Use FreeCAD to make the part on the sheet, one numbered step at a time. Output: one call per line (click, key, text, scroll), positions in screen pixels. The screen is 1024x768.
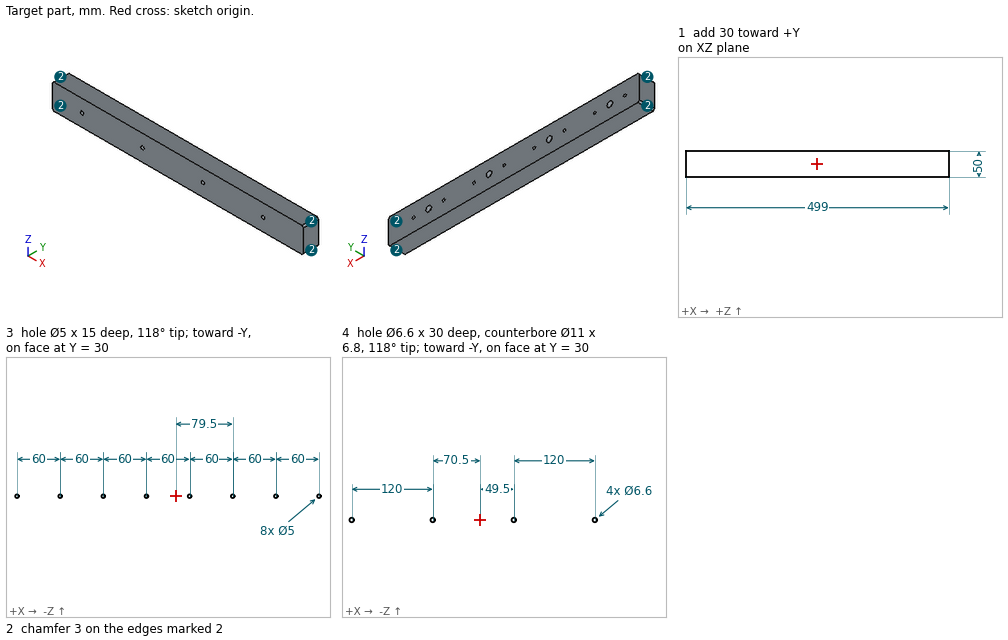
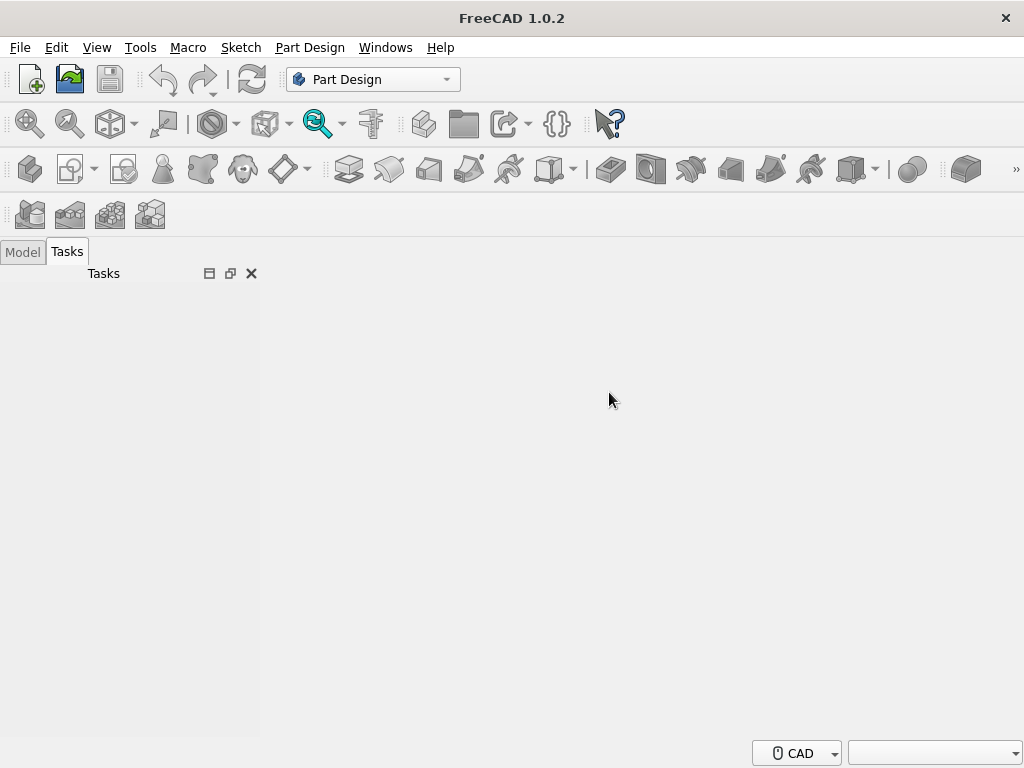
click(30, 80)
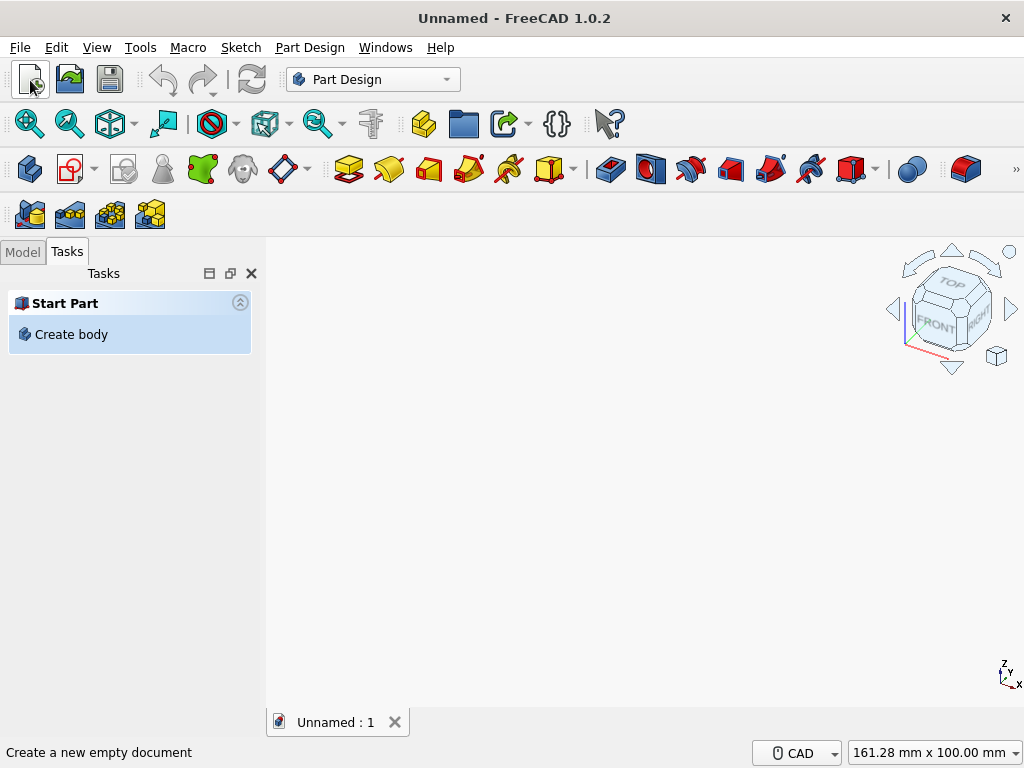
click(70, 170)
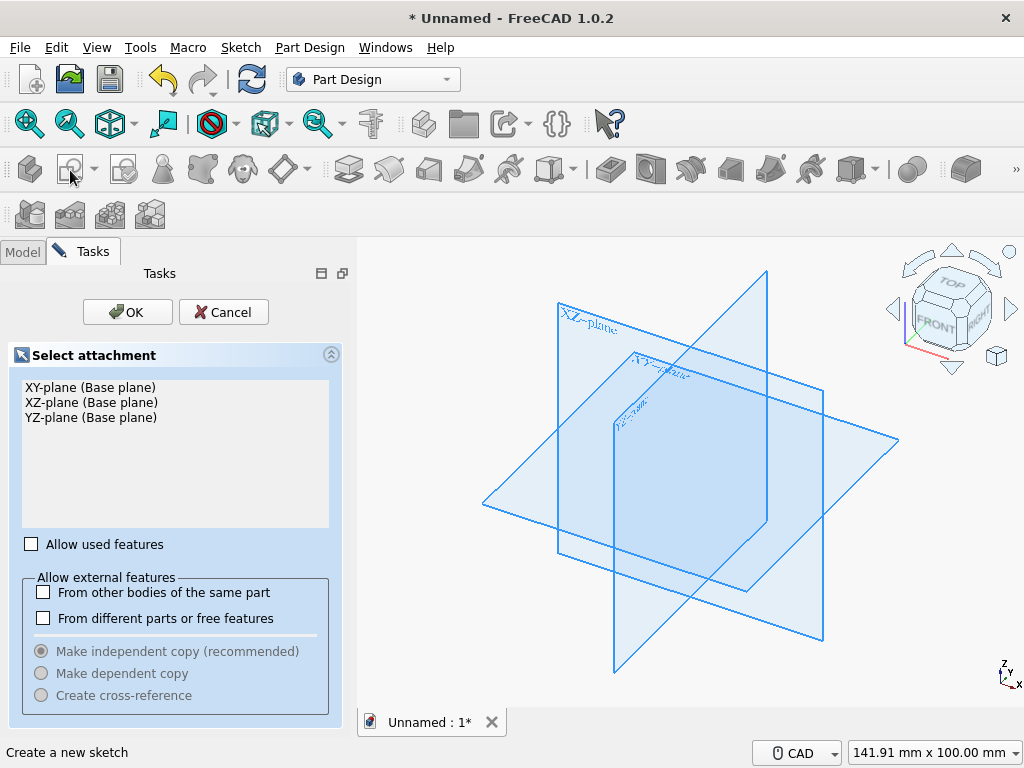
click(82, 402)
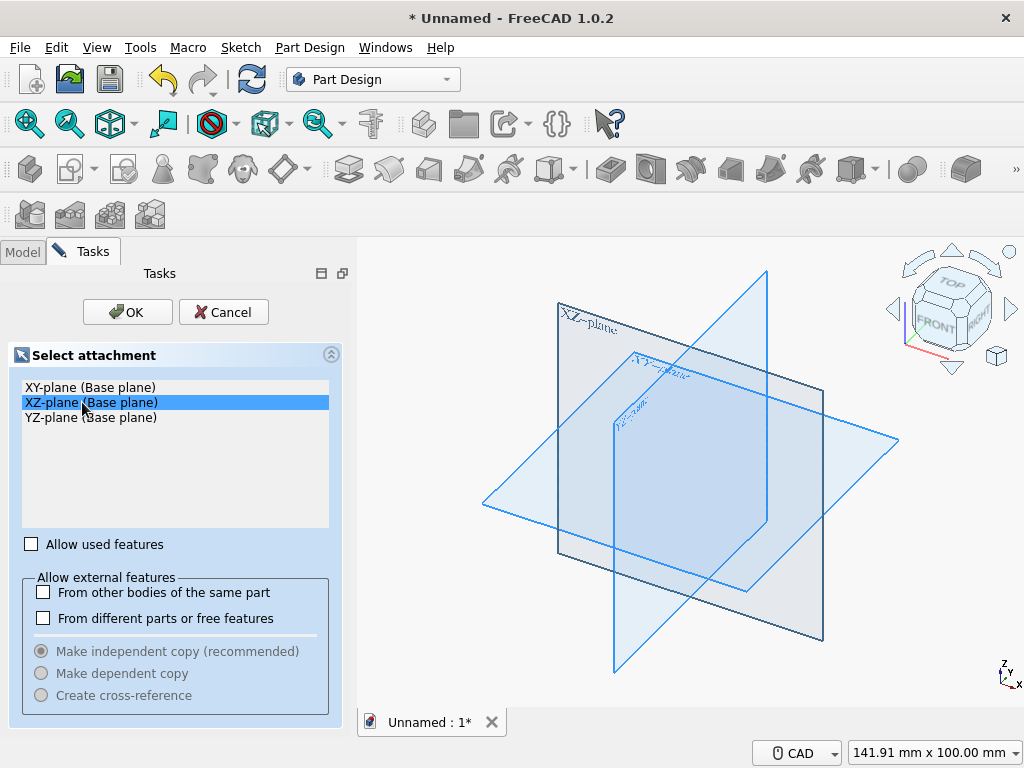
click(128, 312)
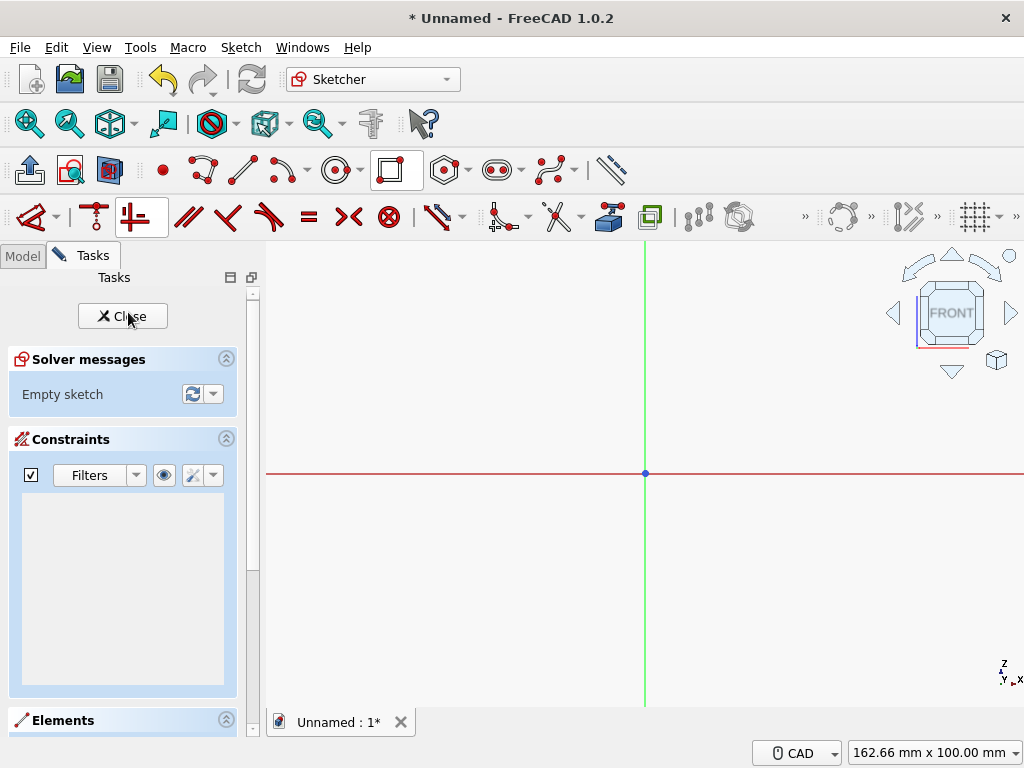
scroll(563, 474, down, 9)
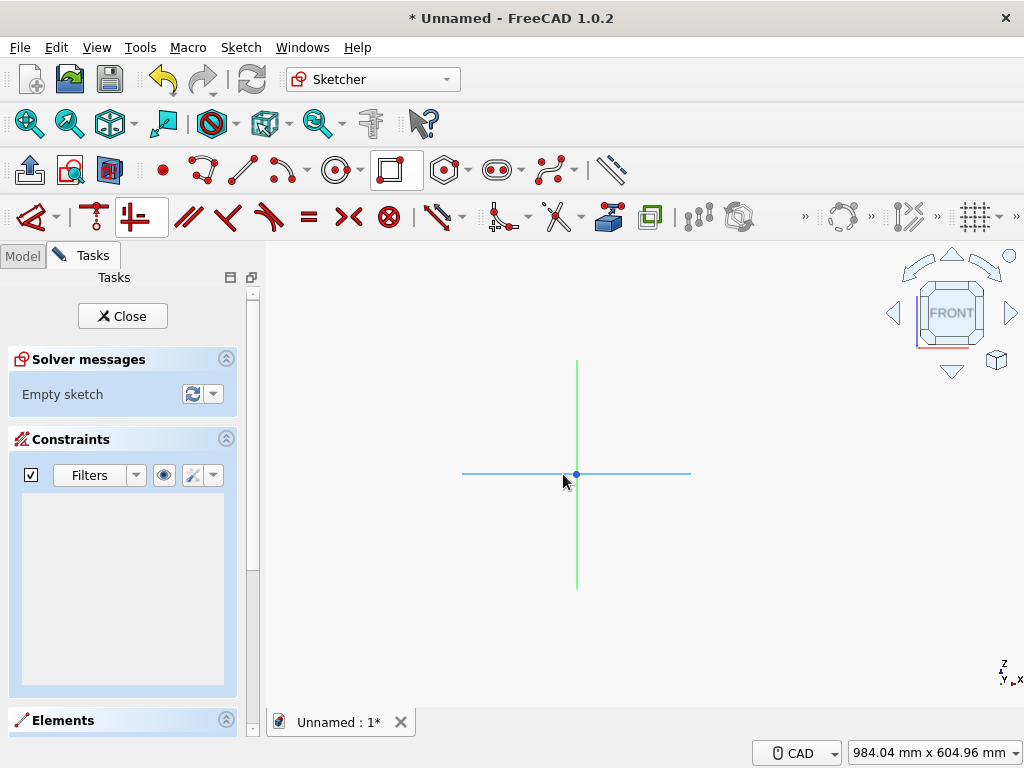
key(g)
key(v)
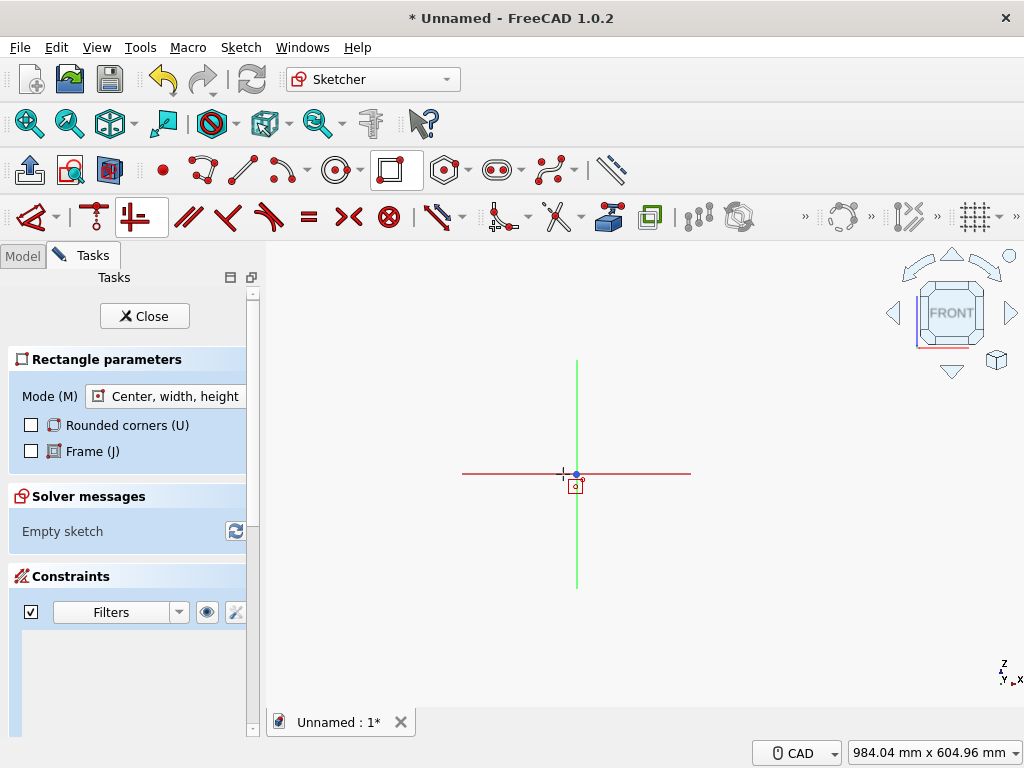
click(577, 474)
click(769, 455)
key(Escape)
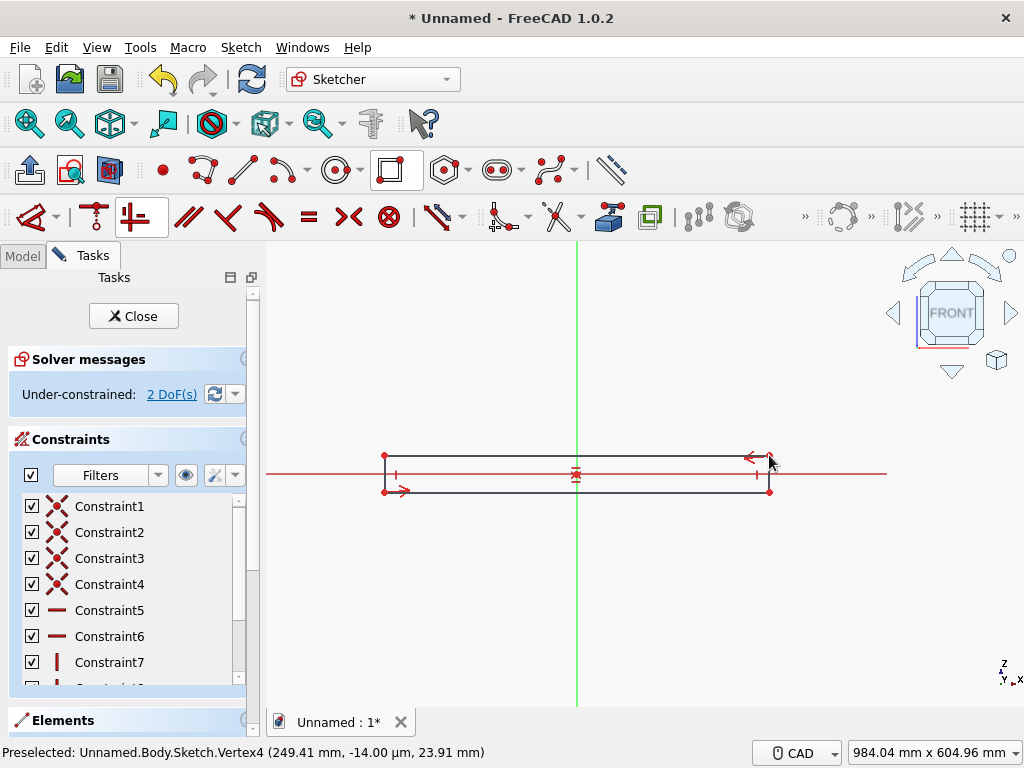
click(32, 218)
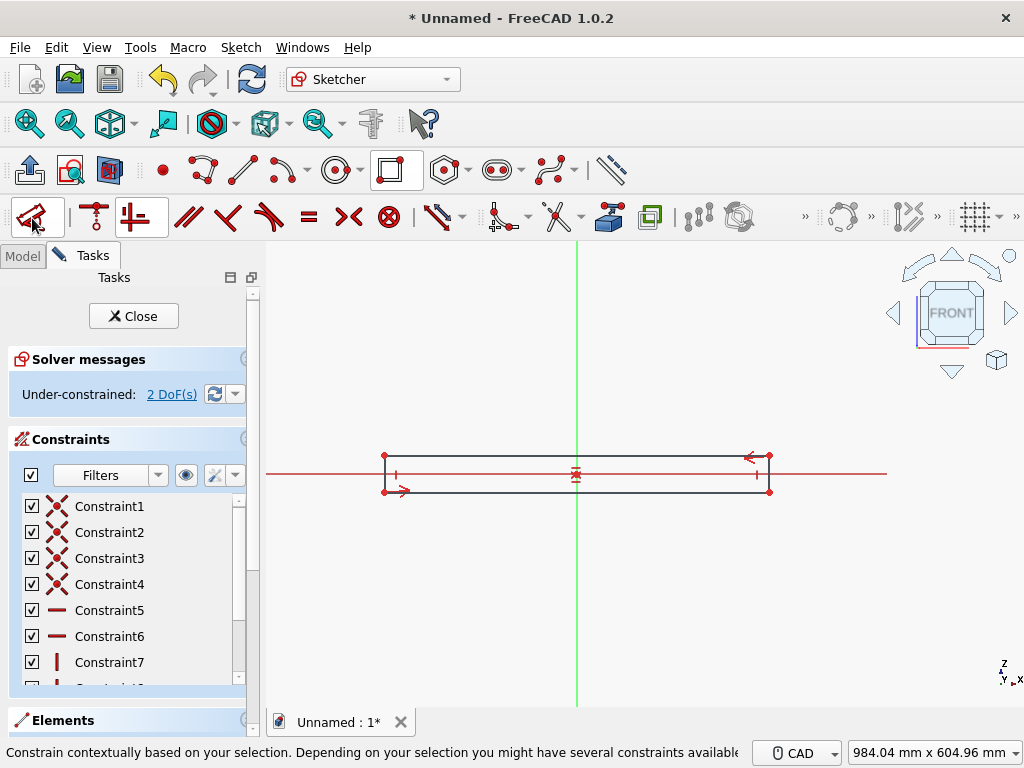
click(769, 478)
click(803, 466)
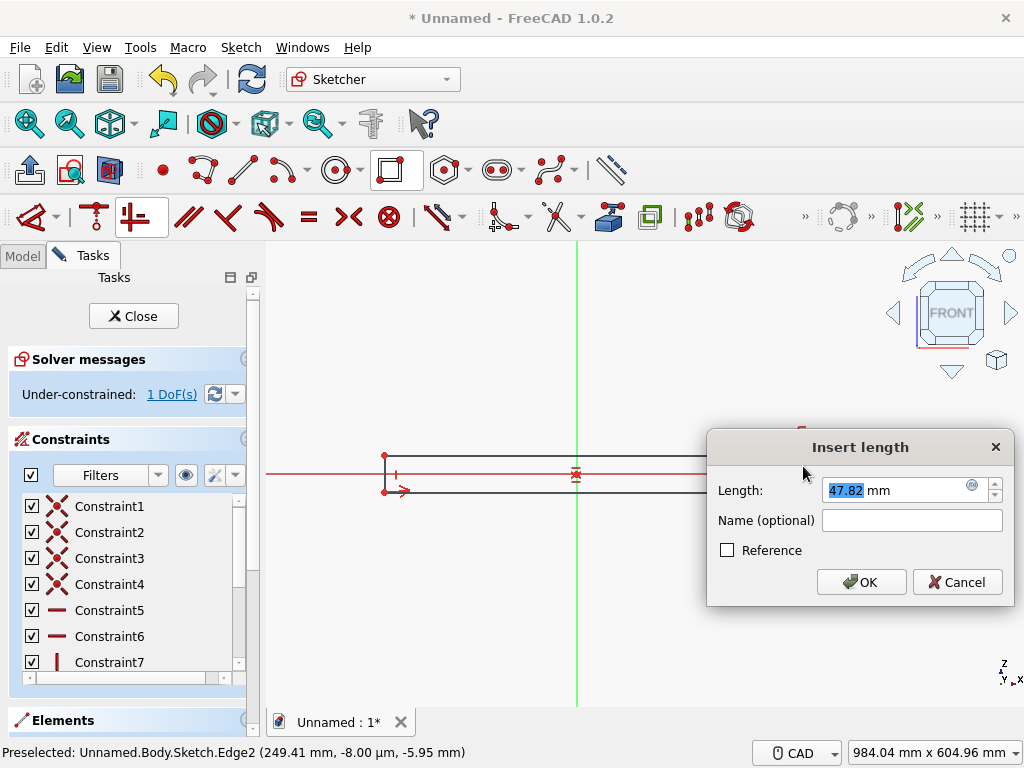
text(50)
key(Return)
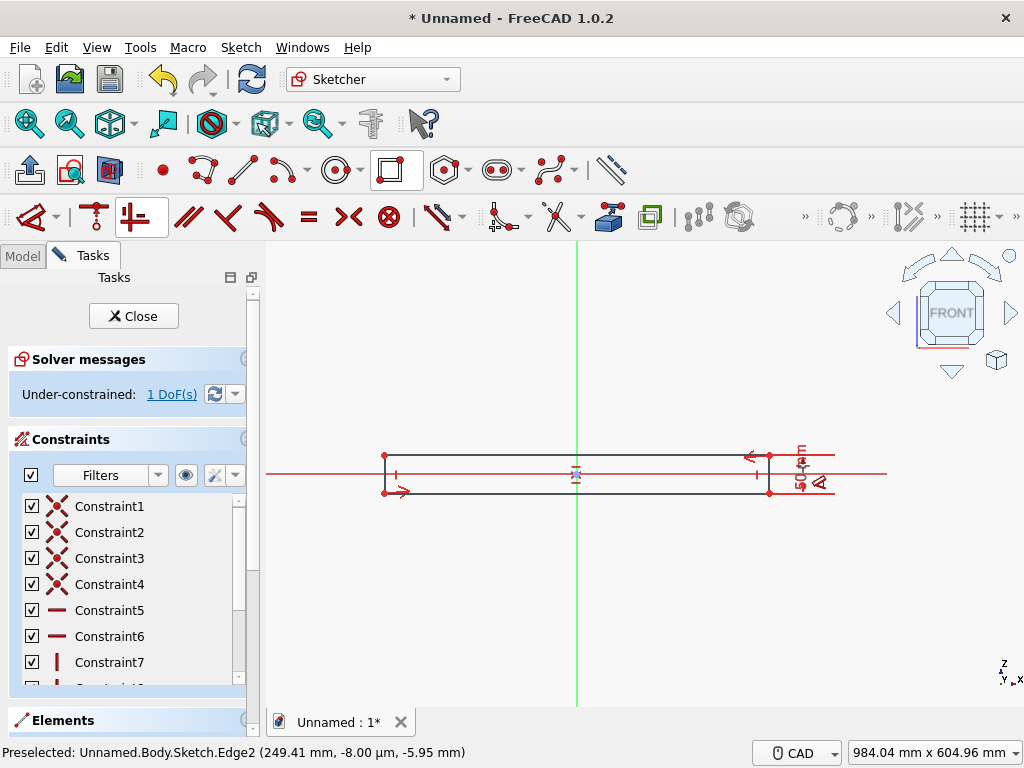
click(500, 494)
click(489, 528)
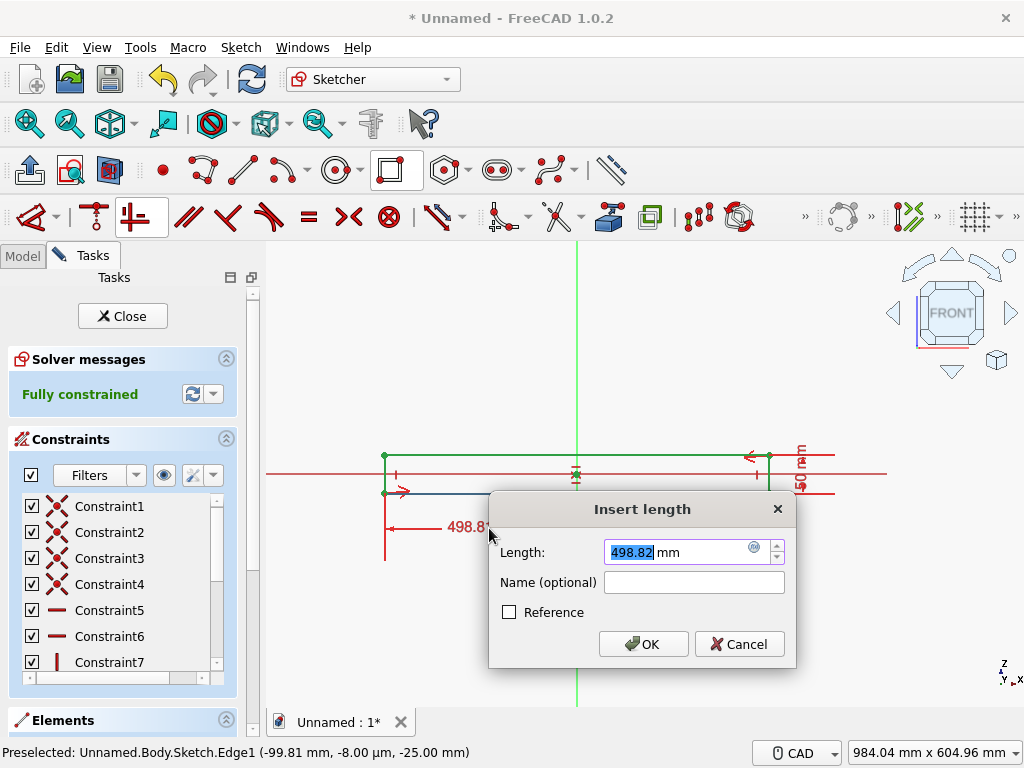
text(499)
key(Return)
key(Escape)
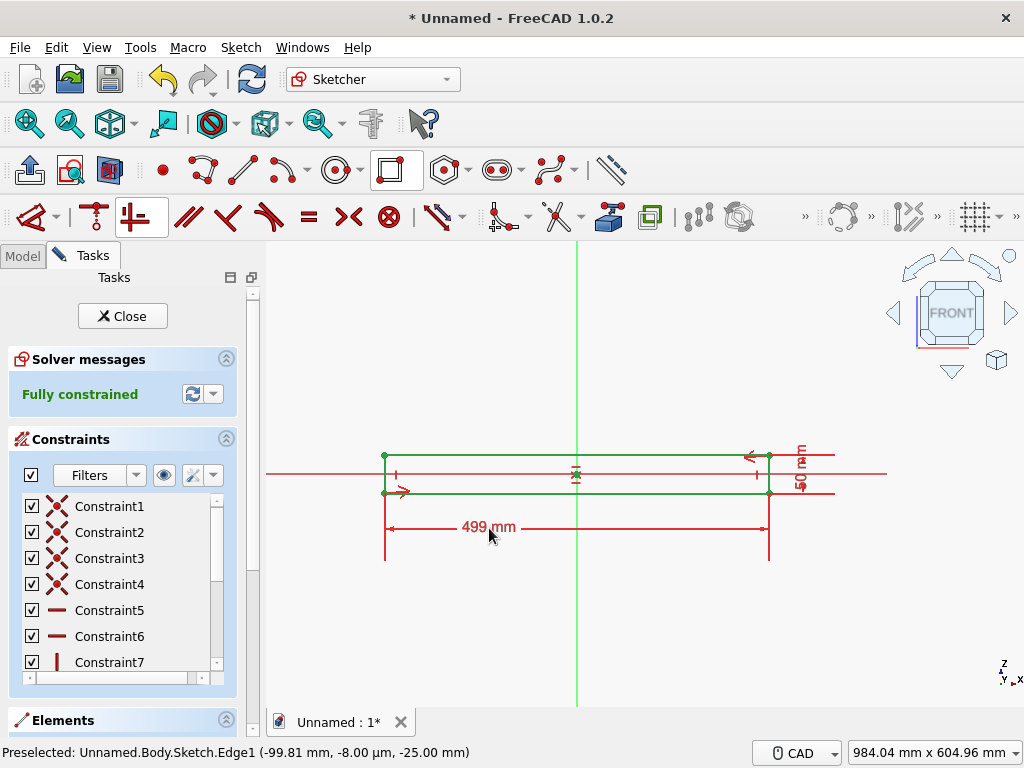
click(123, 316)